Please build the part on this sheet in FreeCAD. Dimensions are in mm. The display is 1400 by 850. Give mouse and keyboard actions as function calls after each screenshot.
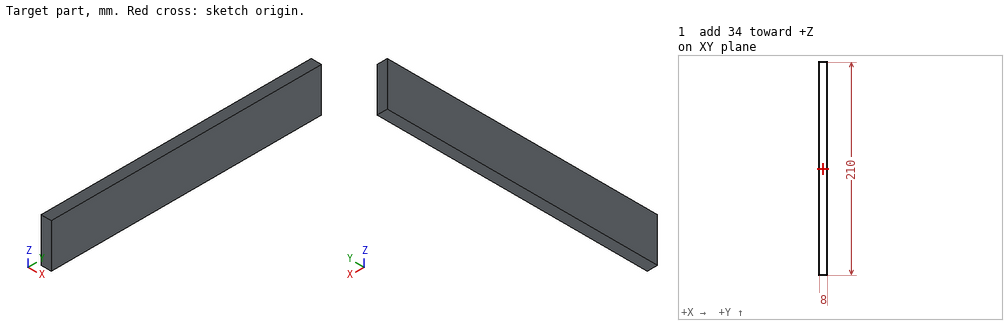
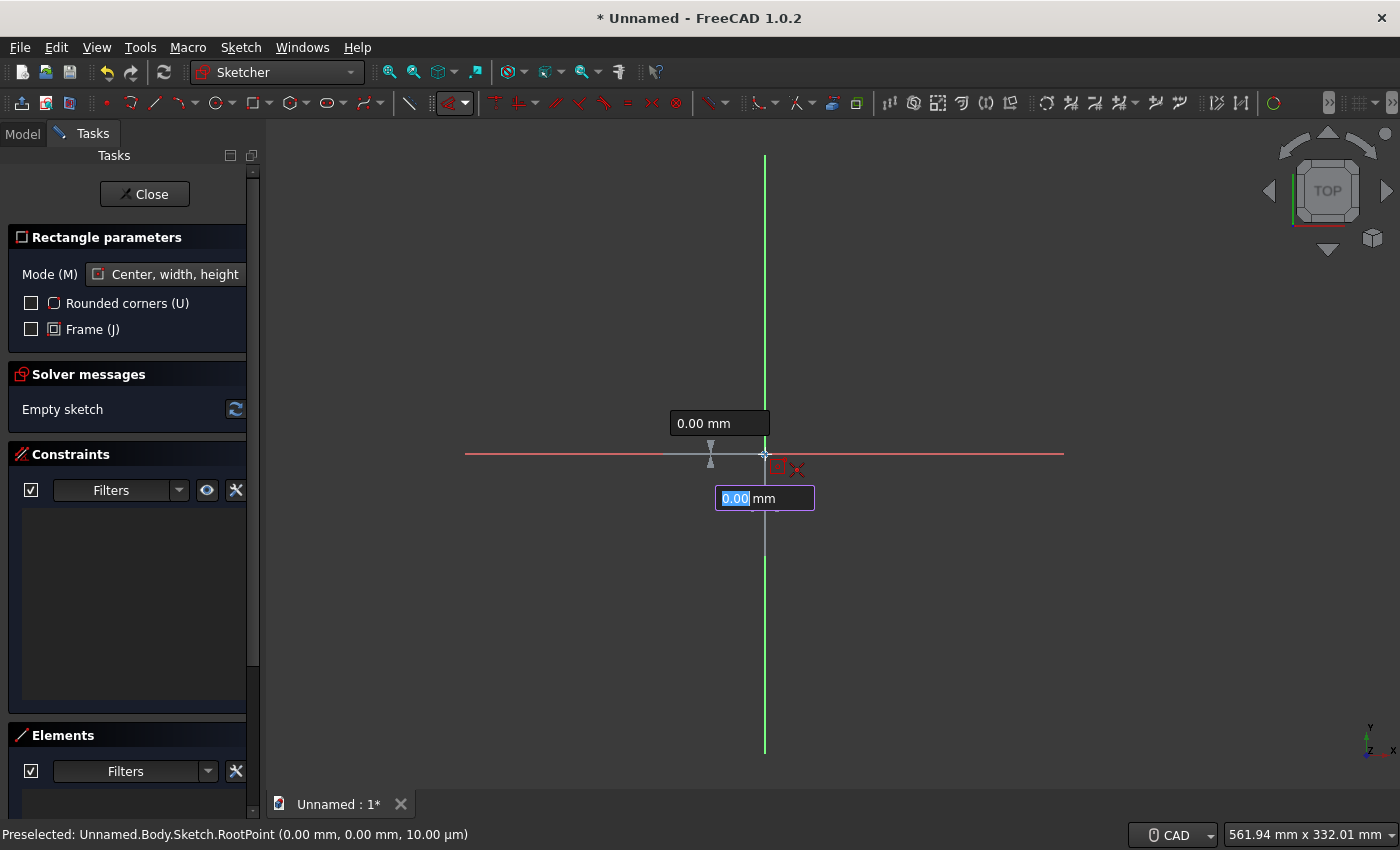
scroll(773, 242, up, 4)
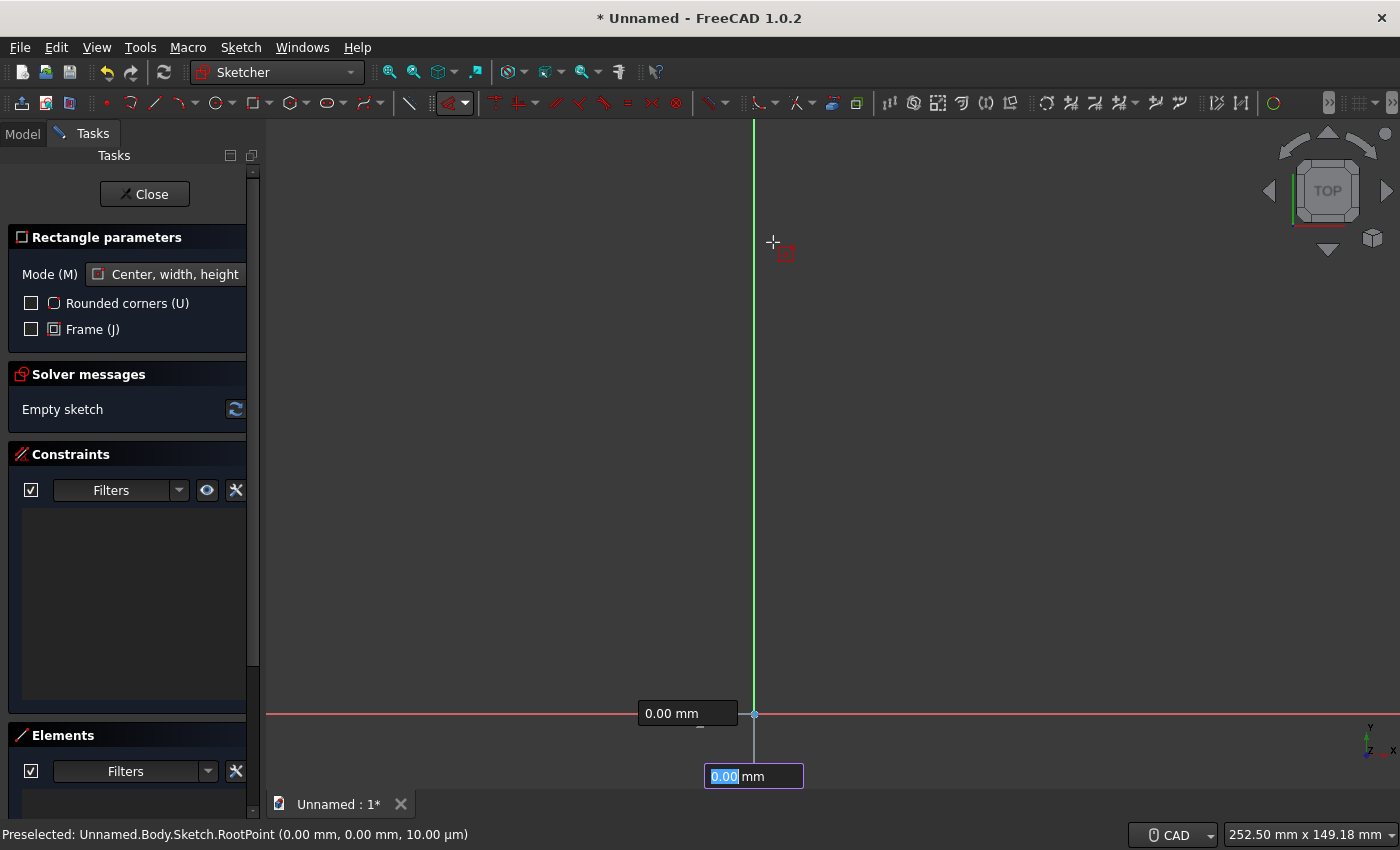
click(772, 243)
key(Escape)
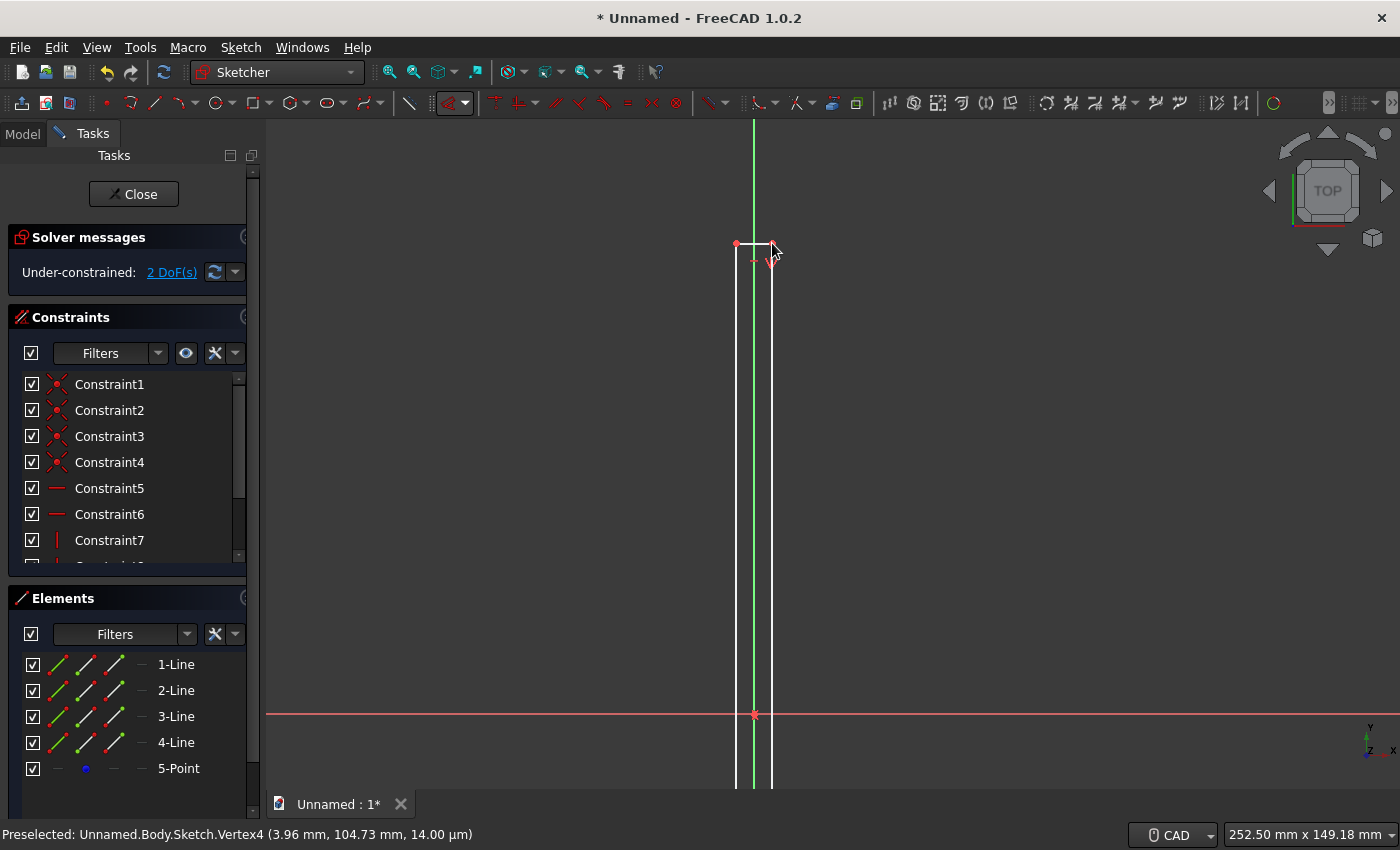
scroll(773, 242, down, 4)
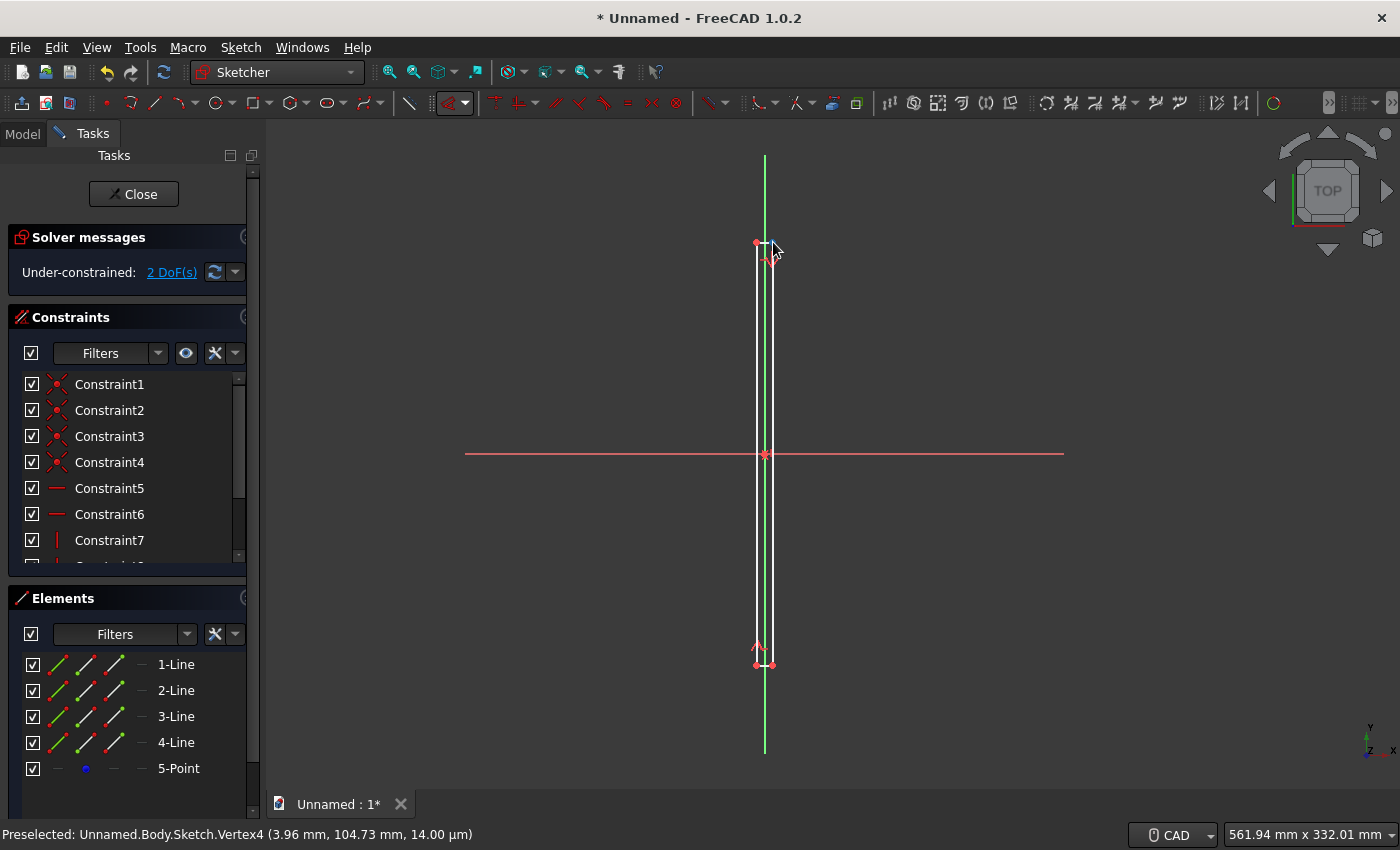
scroll(763, 666, up, 5)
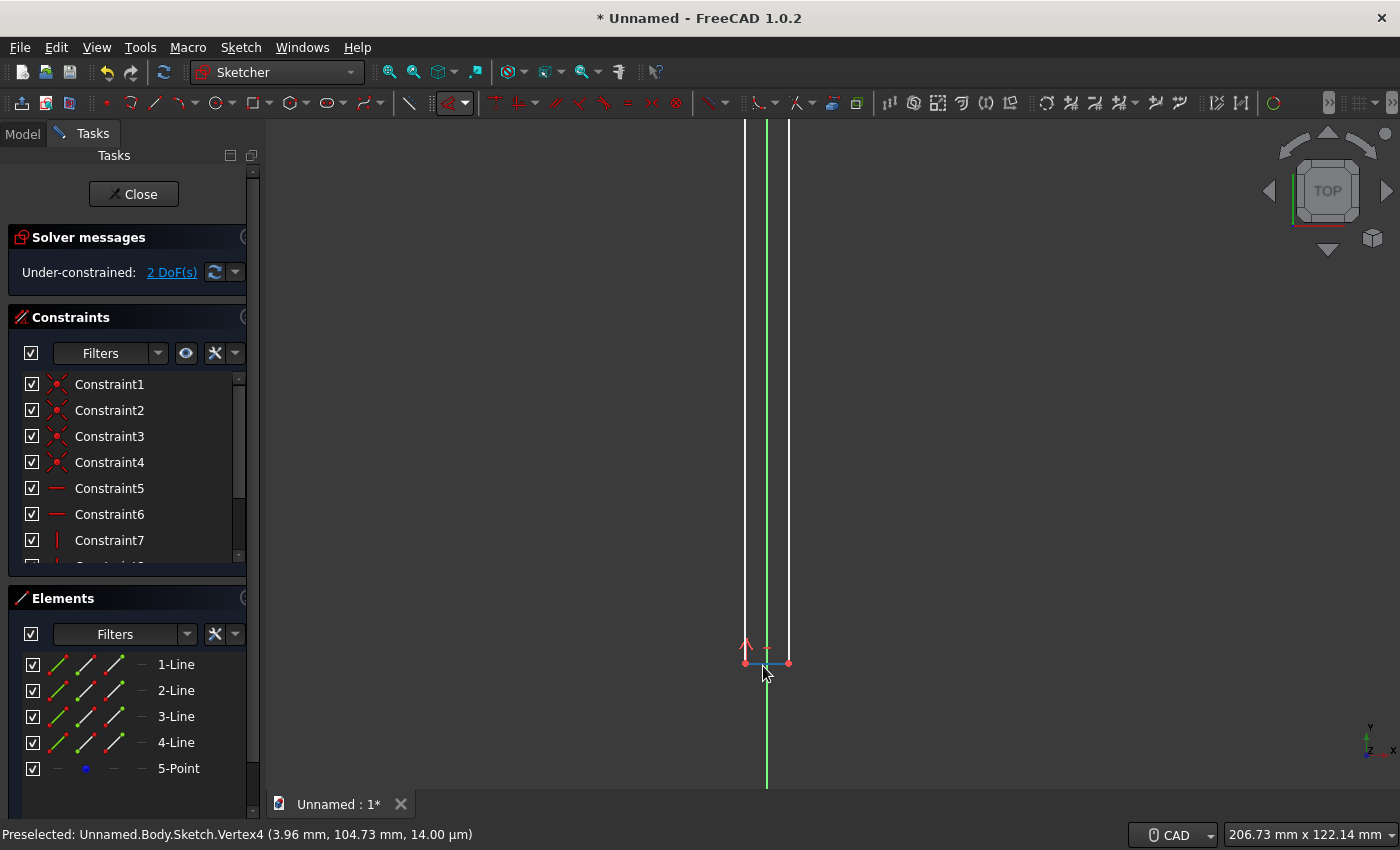
click(763, 664)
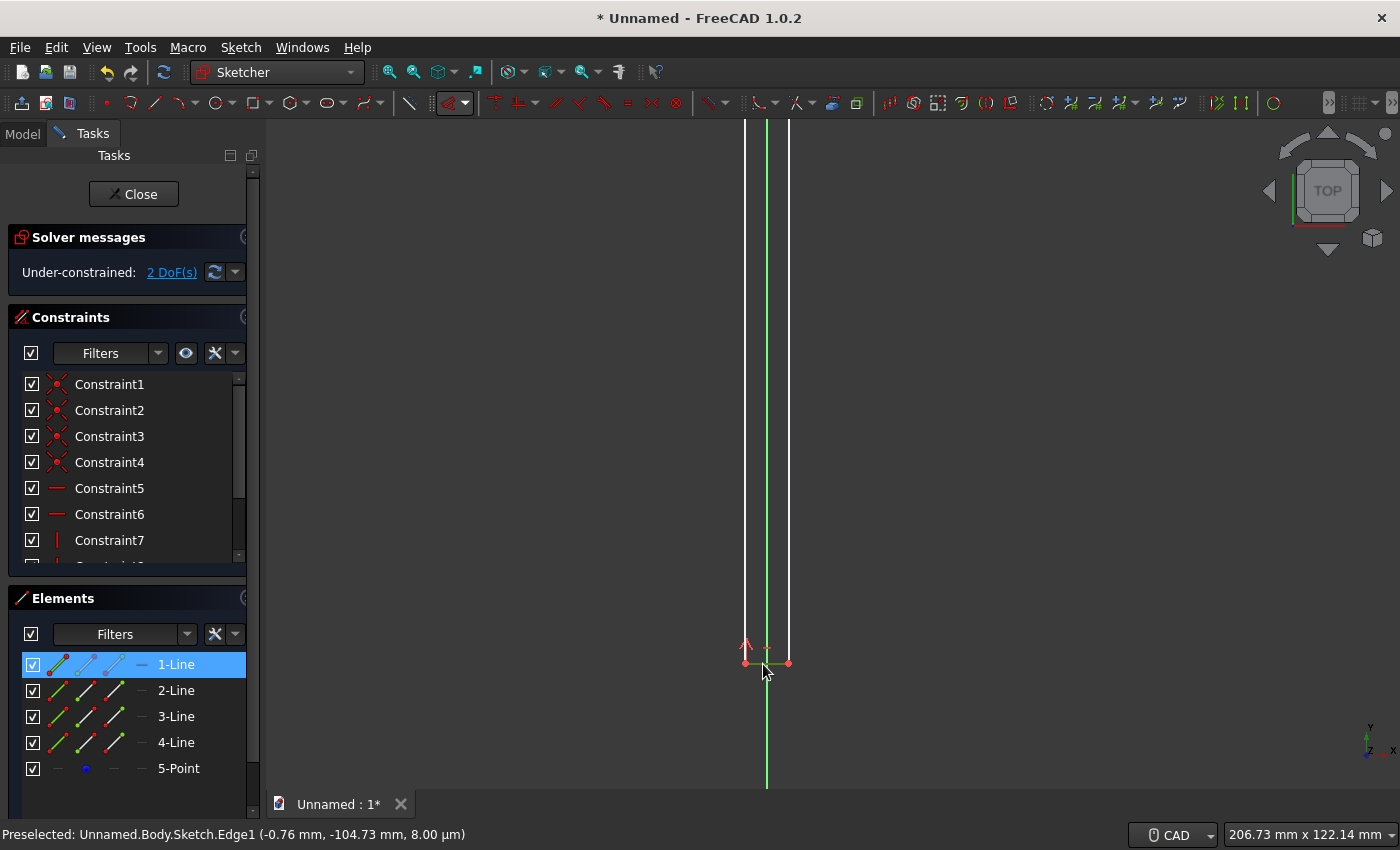
click(468, 104)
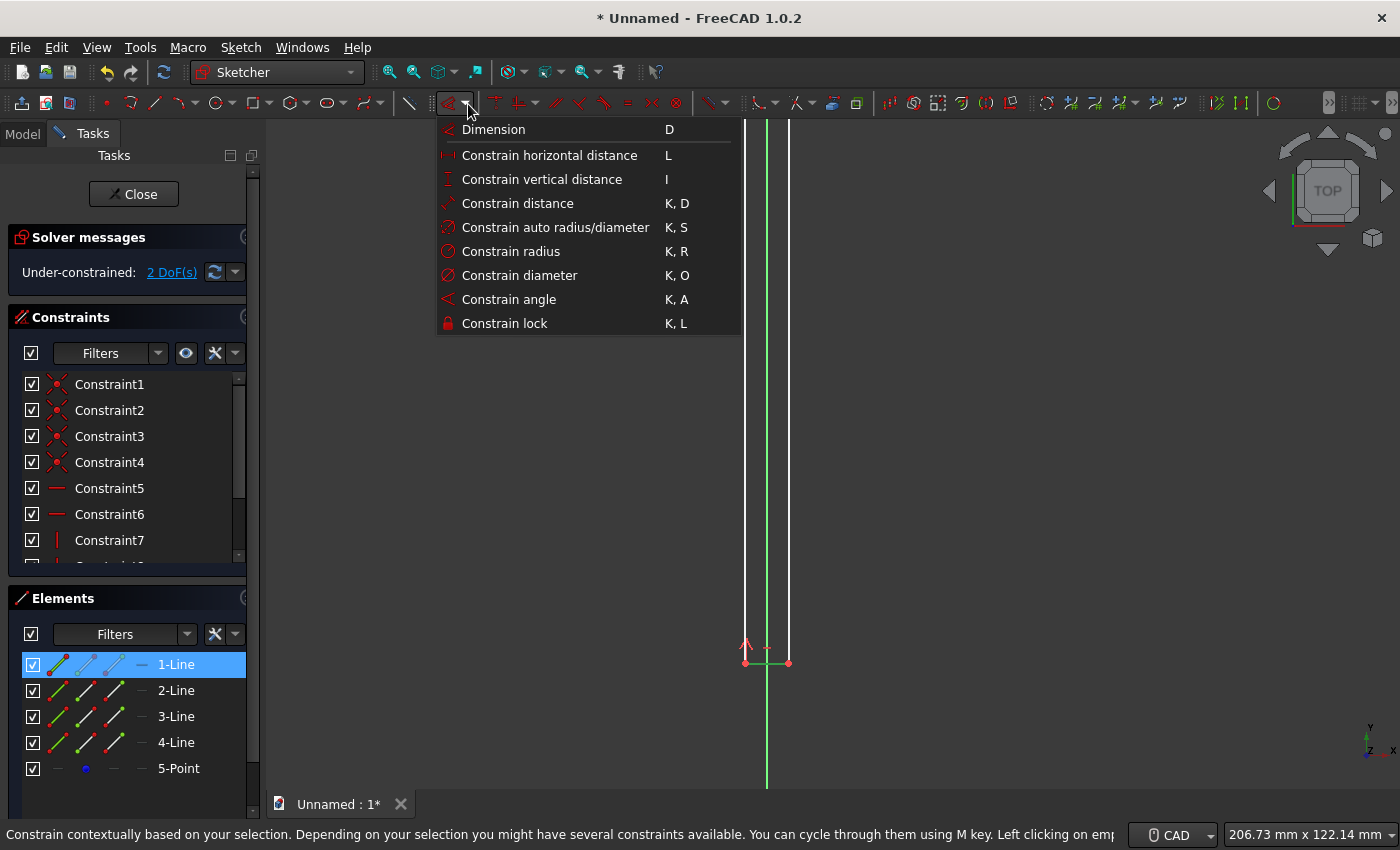
click(589, 155)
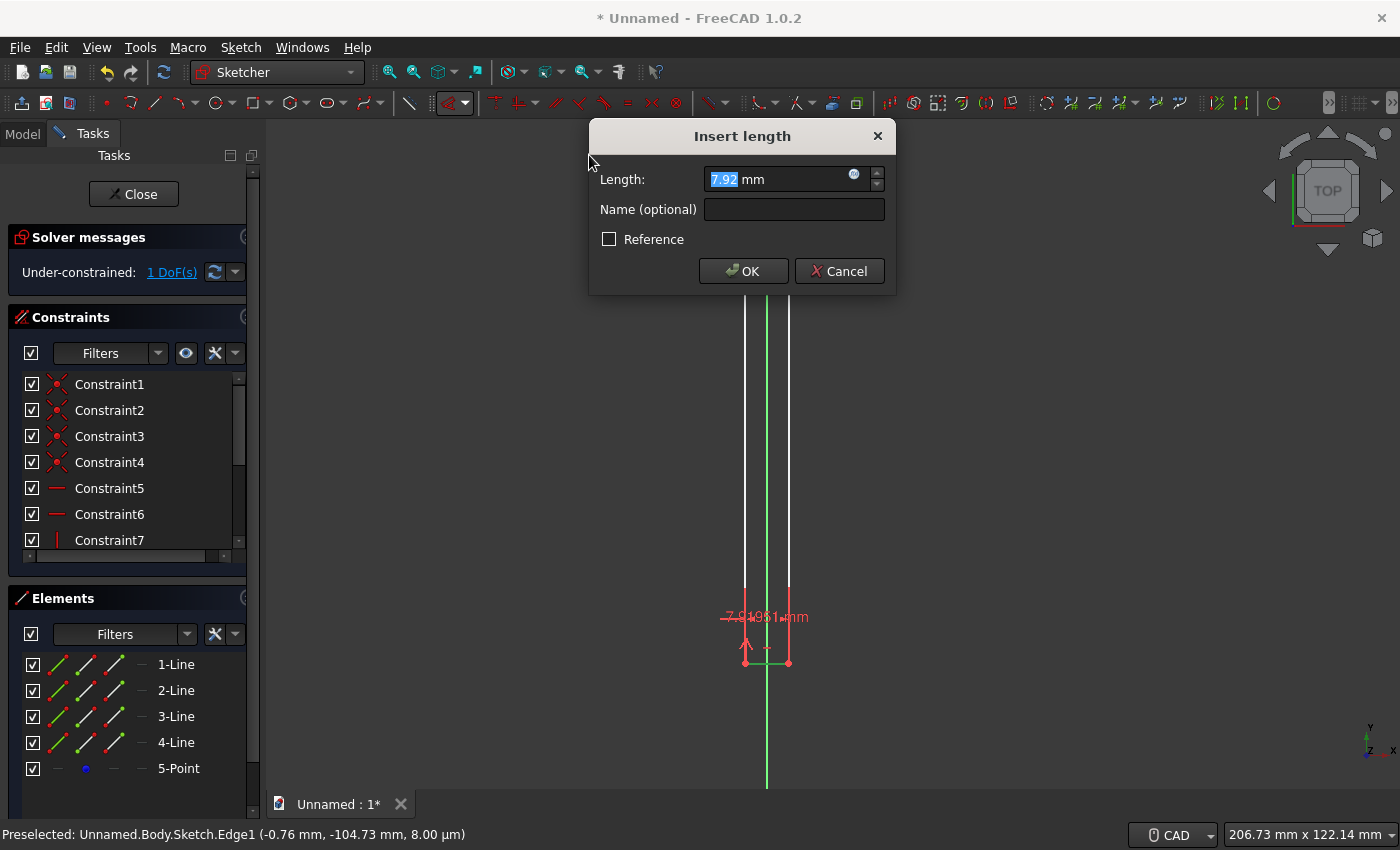
text(8)
key(Return)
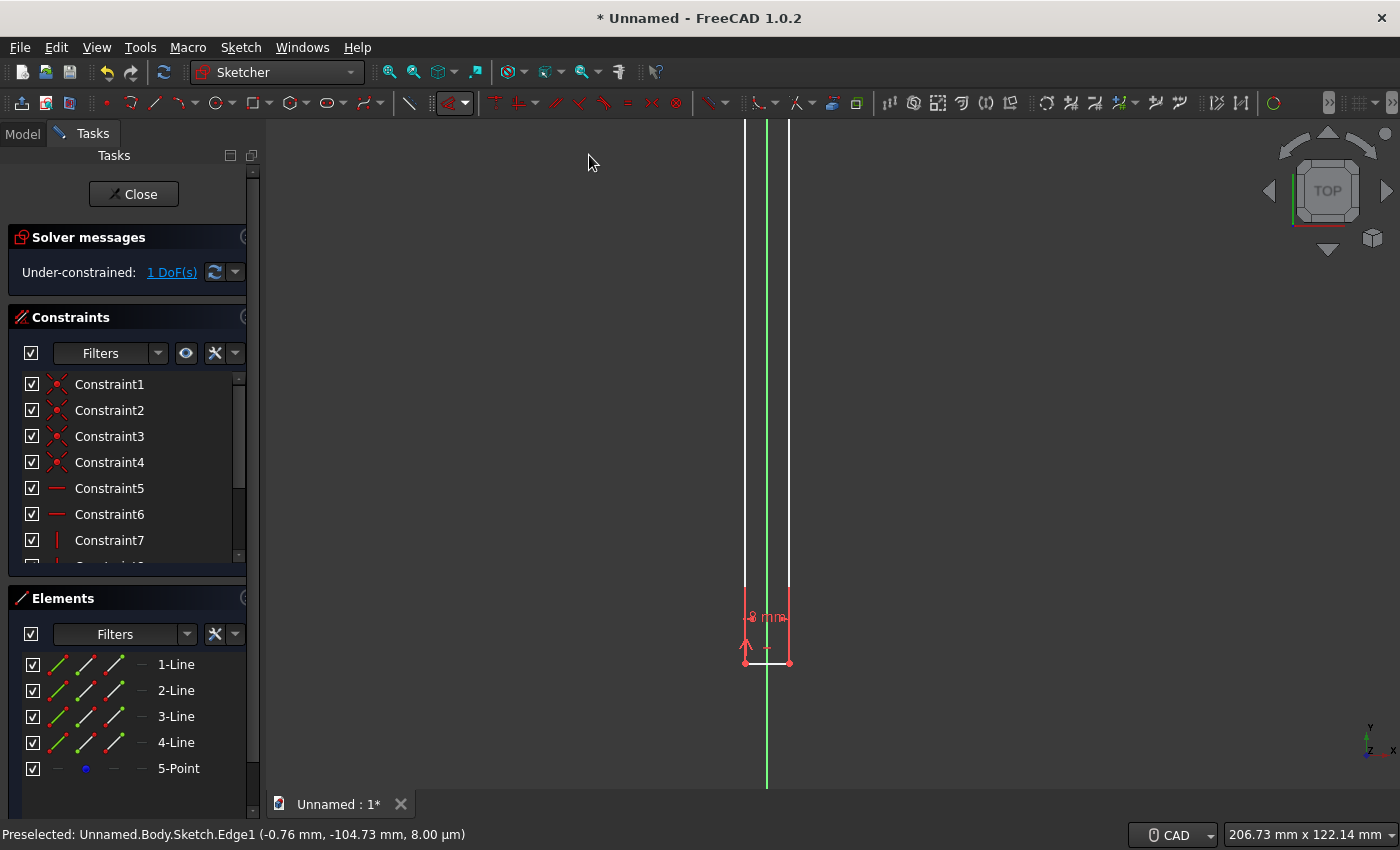
click(789, 319)